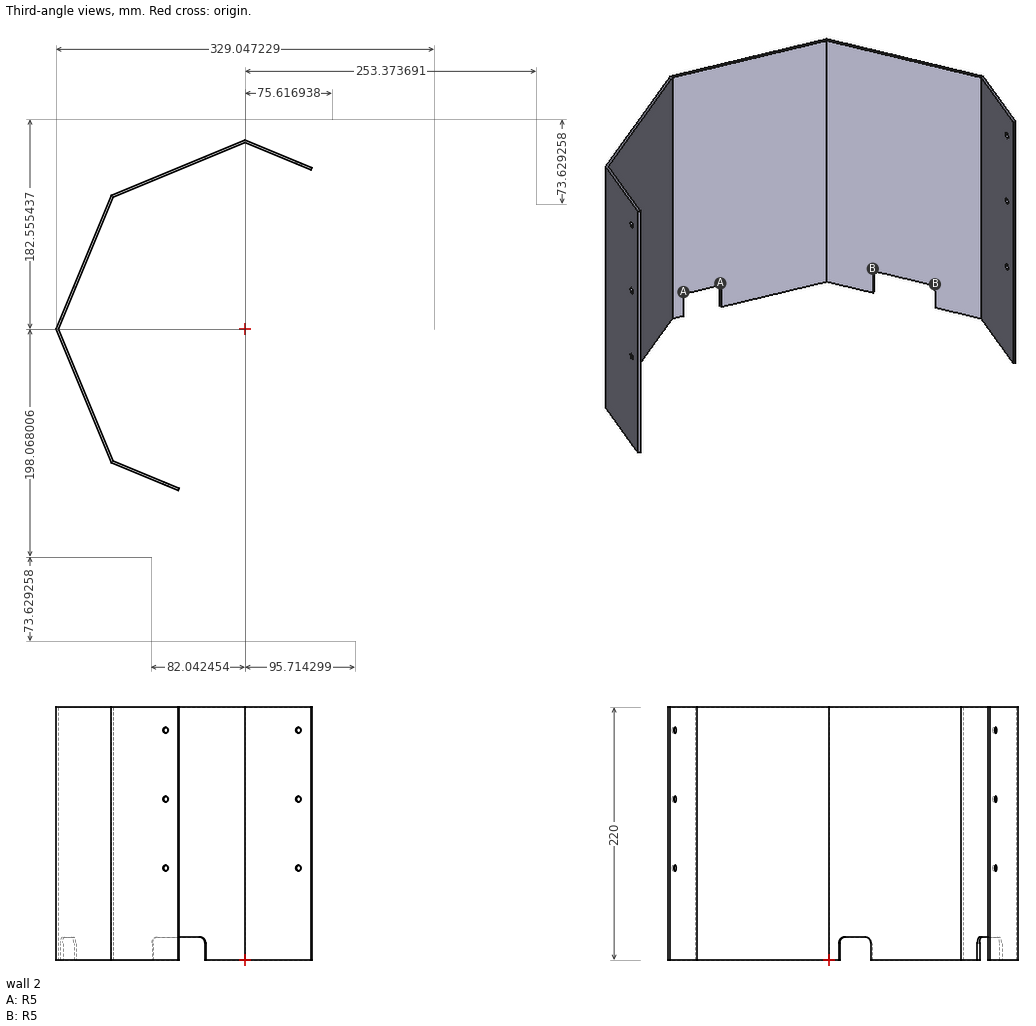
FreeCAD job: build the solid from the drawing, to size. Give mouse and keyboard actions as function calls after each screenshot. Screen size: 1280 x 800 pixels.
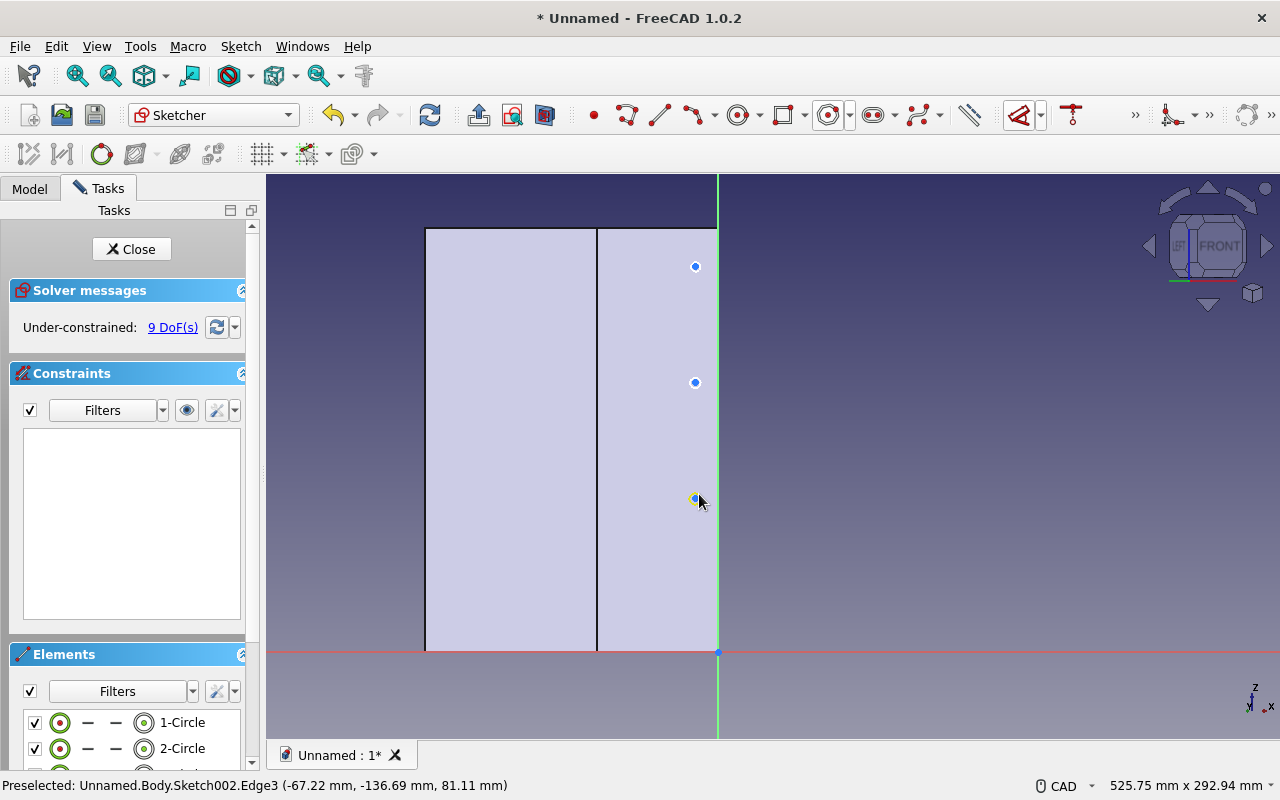
scroll(699, 264, up, 6)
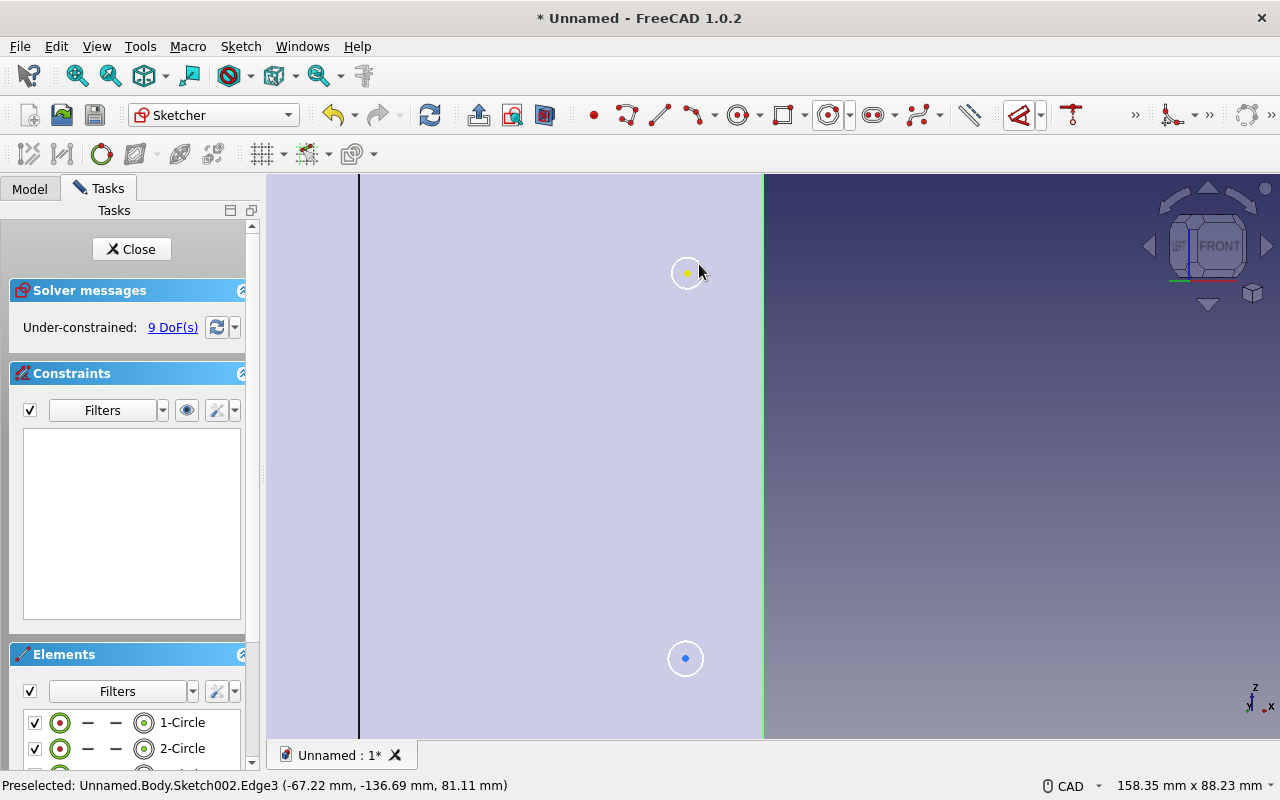
click(698, 262)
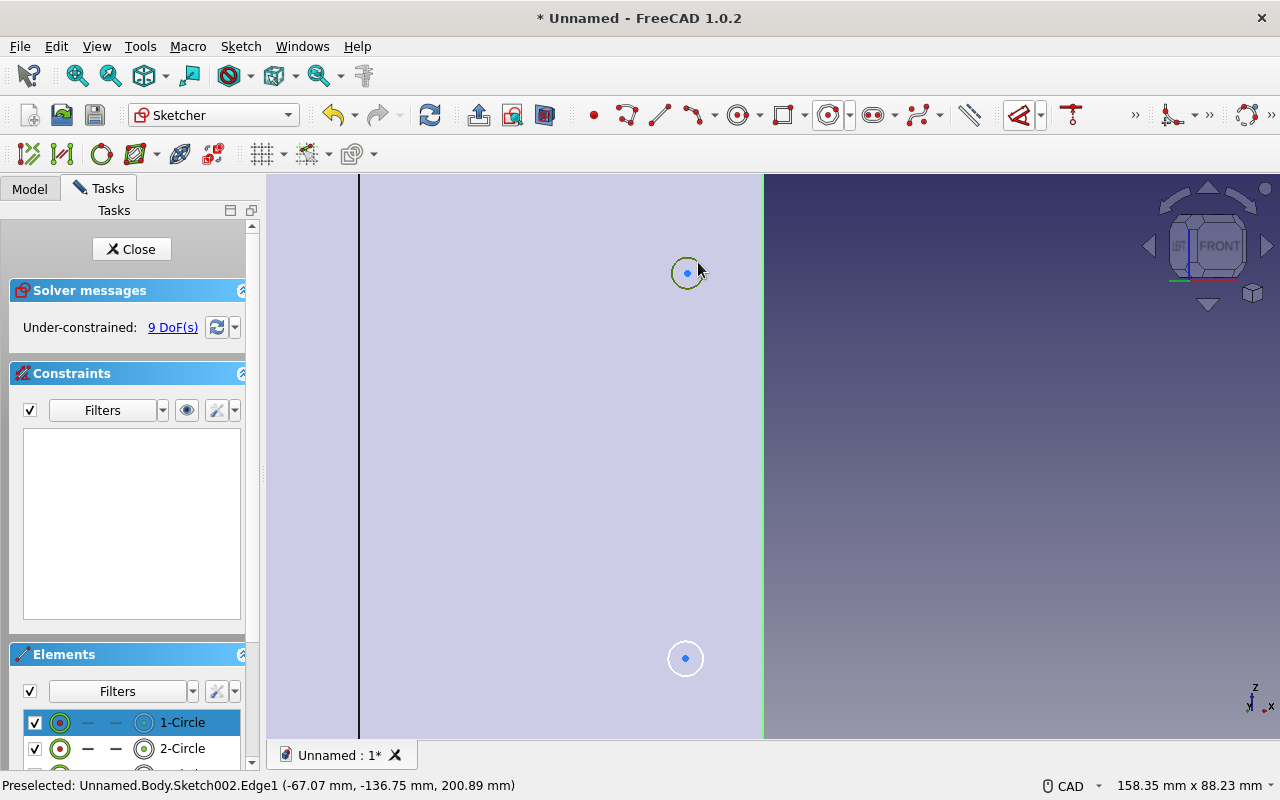
click(698, 646)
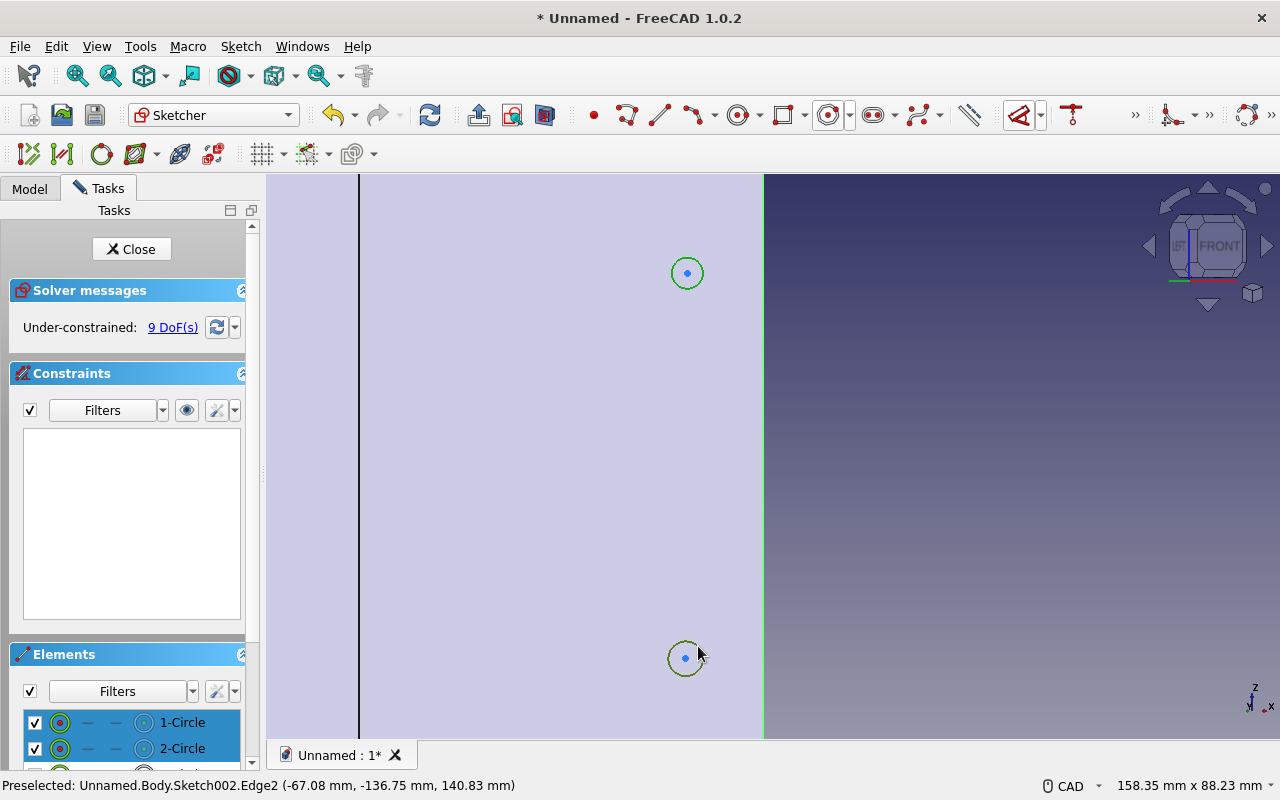
scroll(699, 264, down, 6)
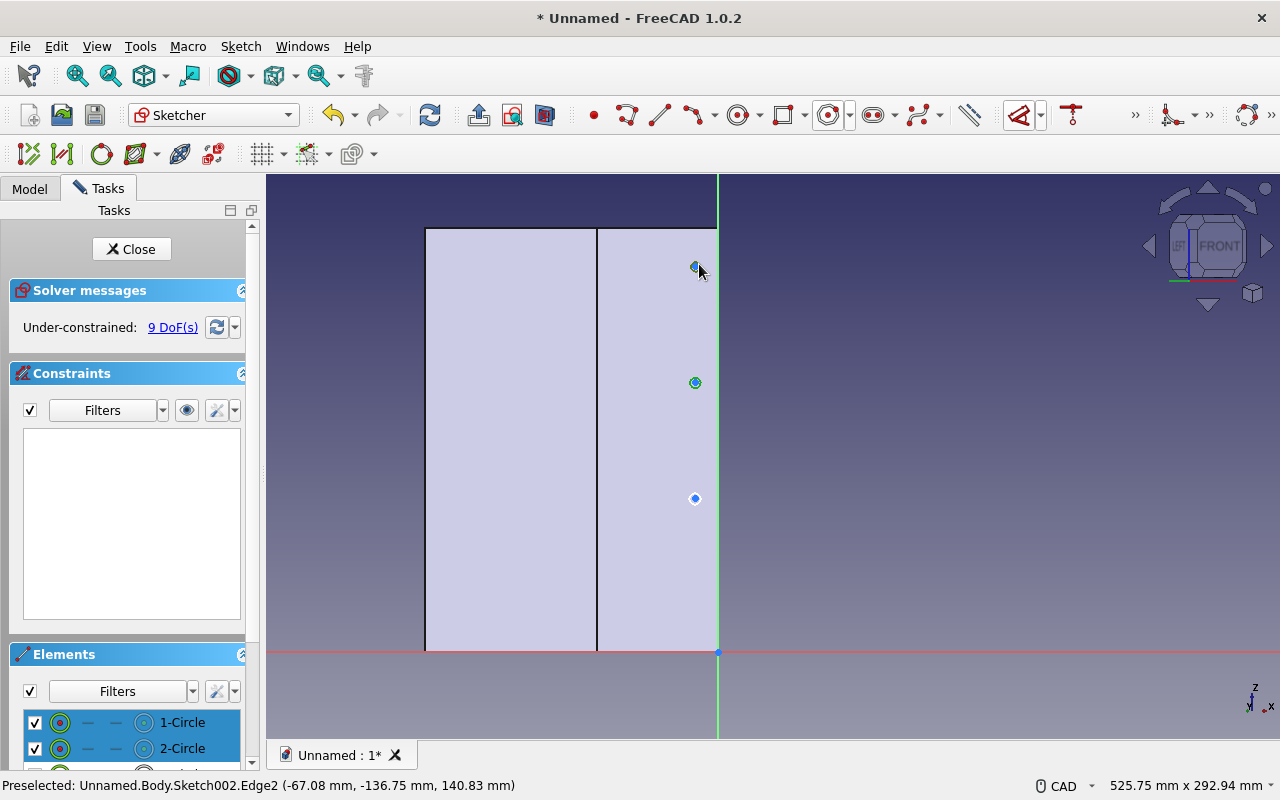
scroll(699, 495, up, 5)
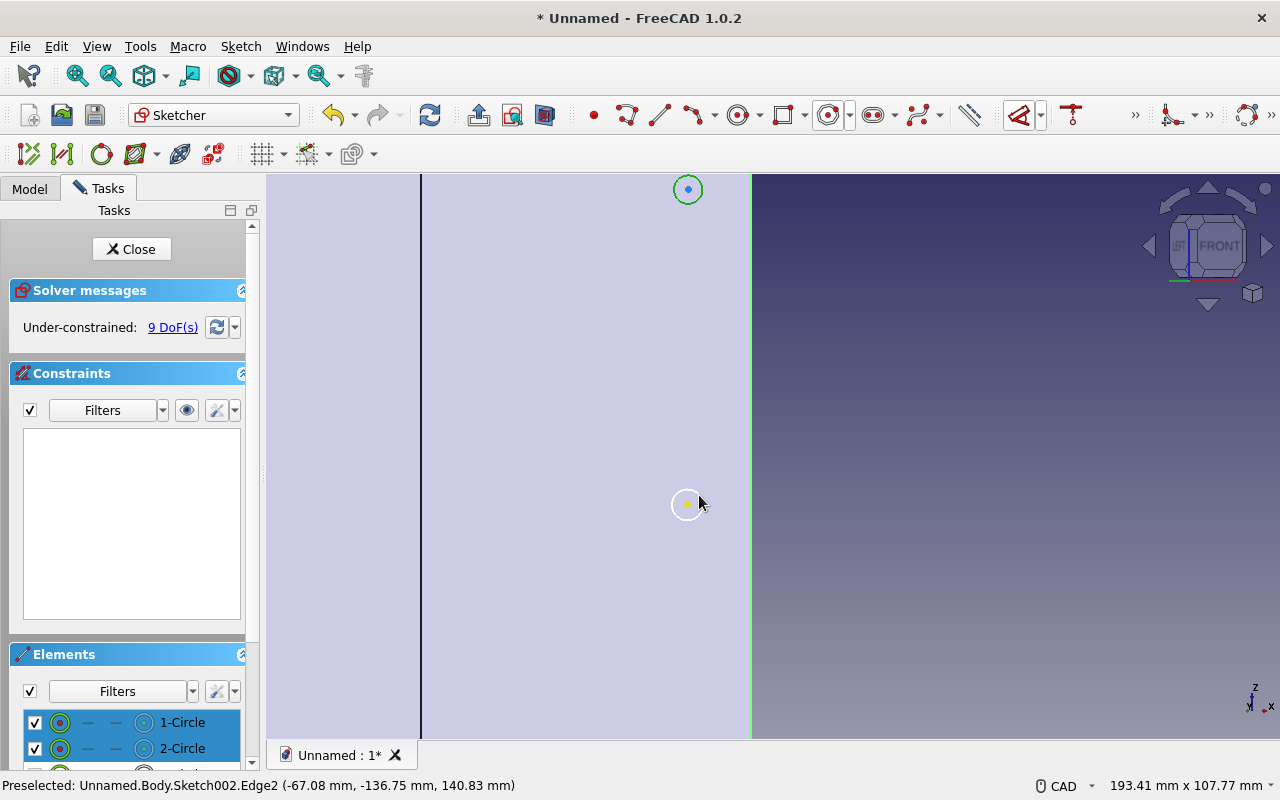
click(698, 494)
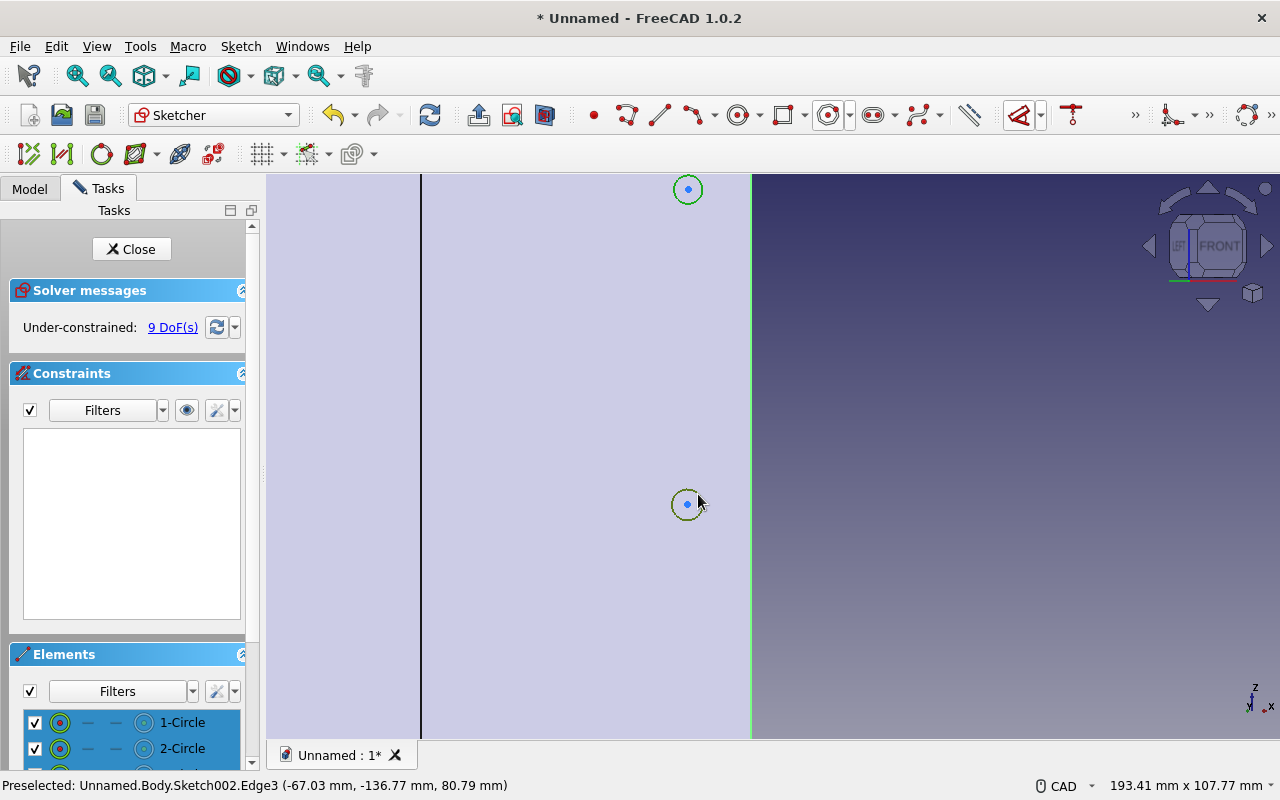
key(e)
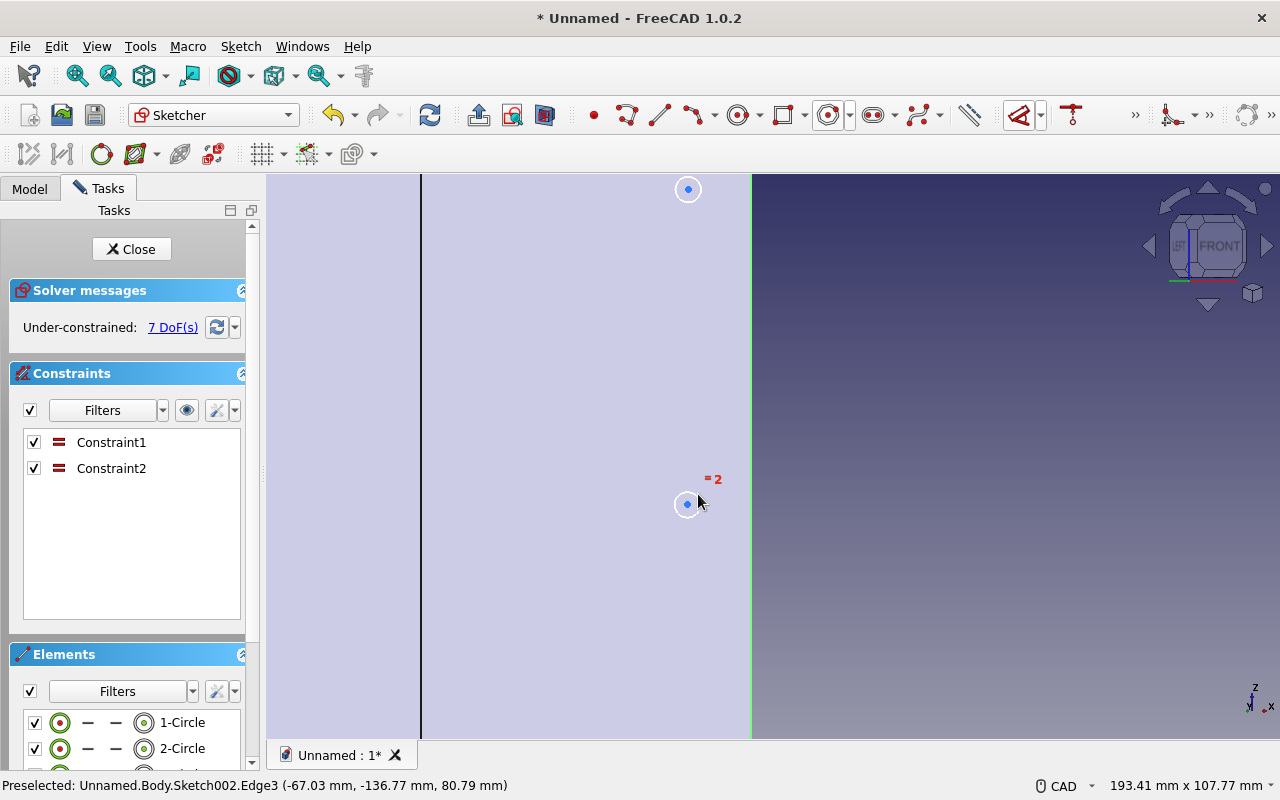
scroll(699, 495, down, 5)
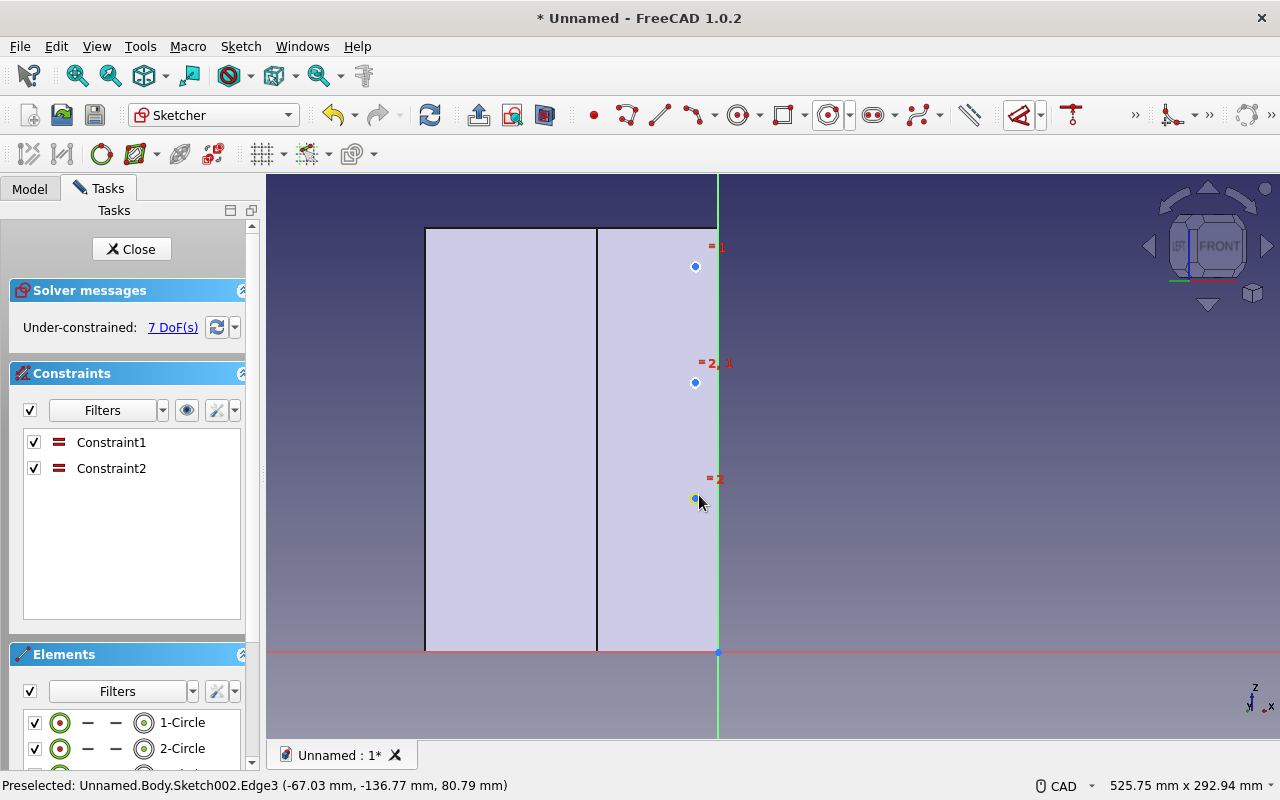
click(696, 267)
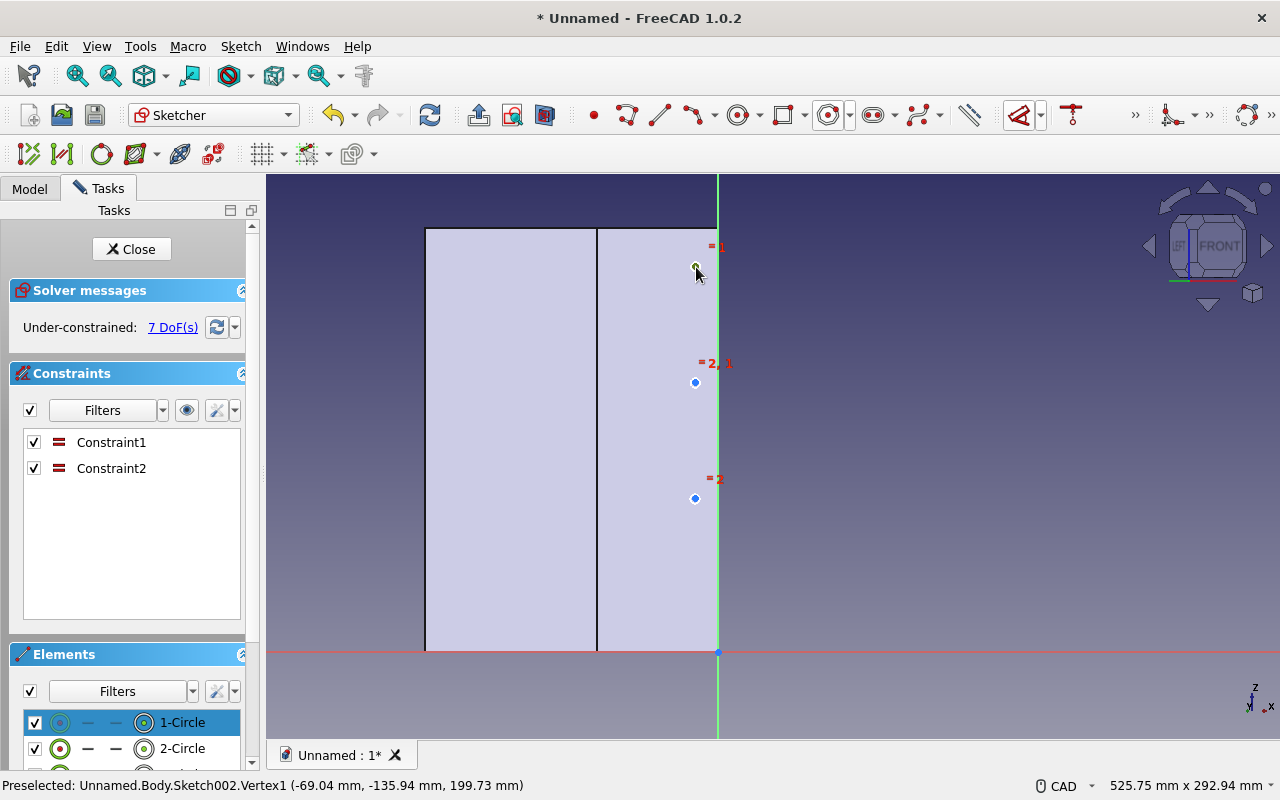
click(695, 383)